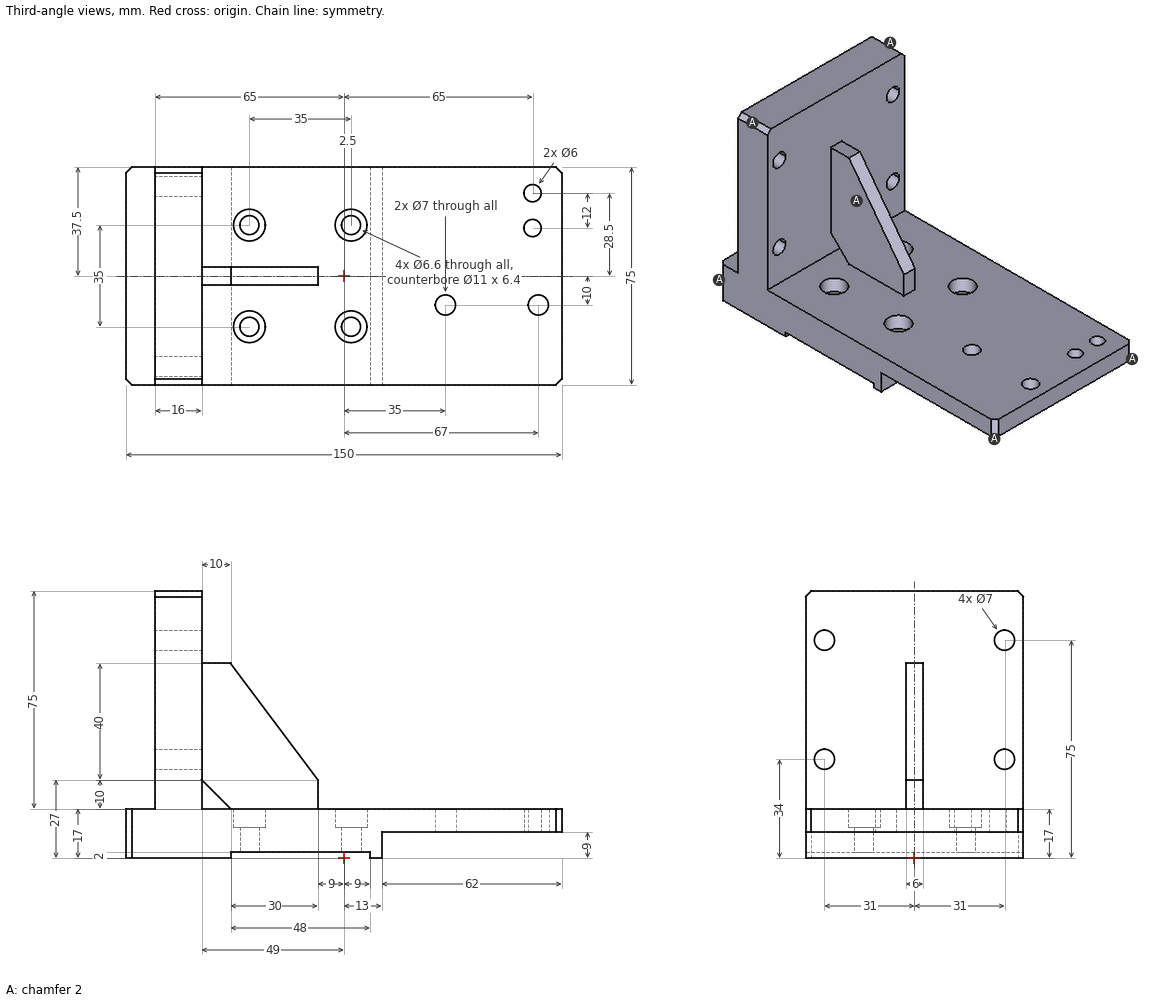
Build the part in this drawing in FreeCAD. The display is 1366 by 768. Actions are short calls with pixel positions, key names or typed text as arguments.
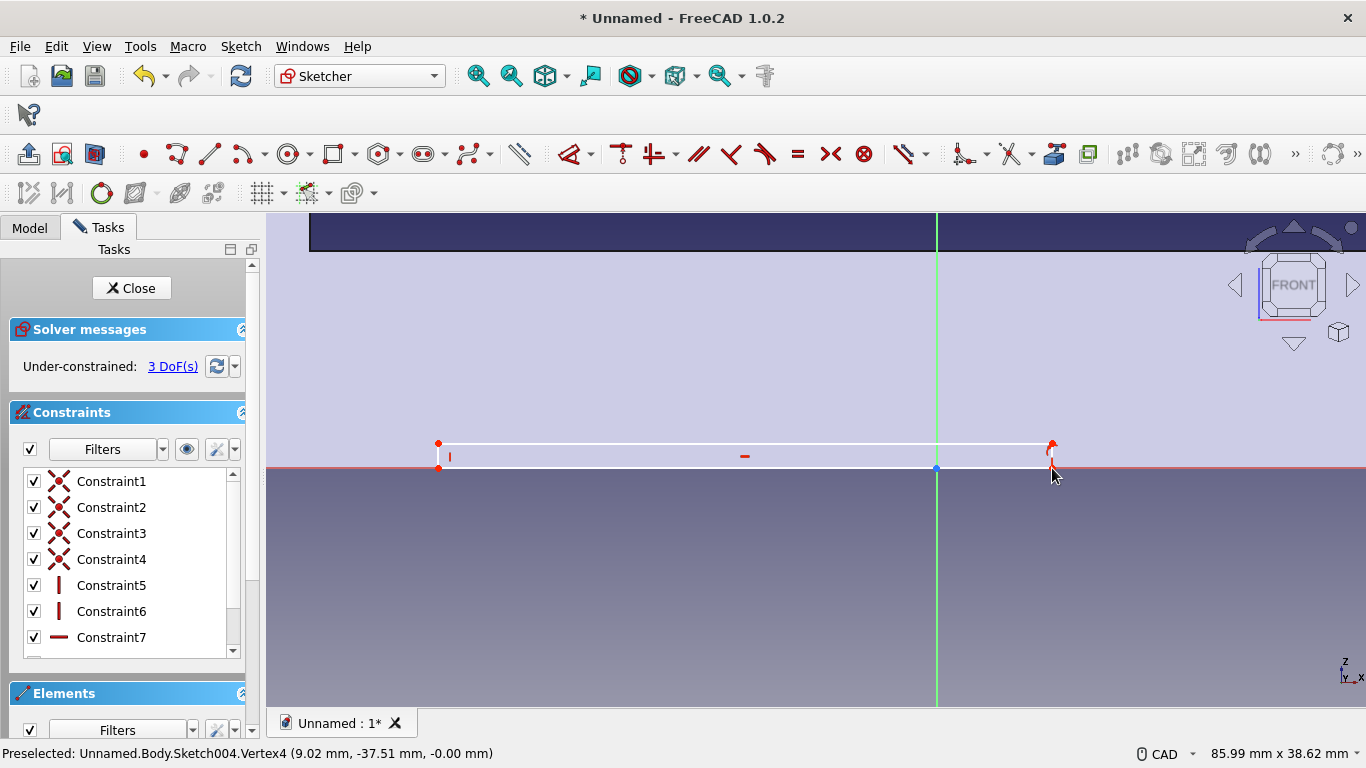
click(568, 154)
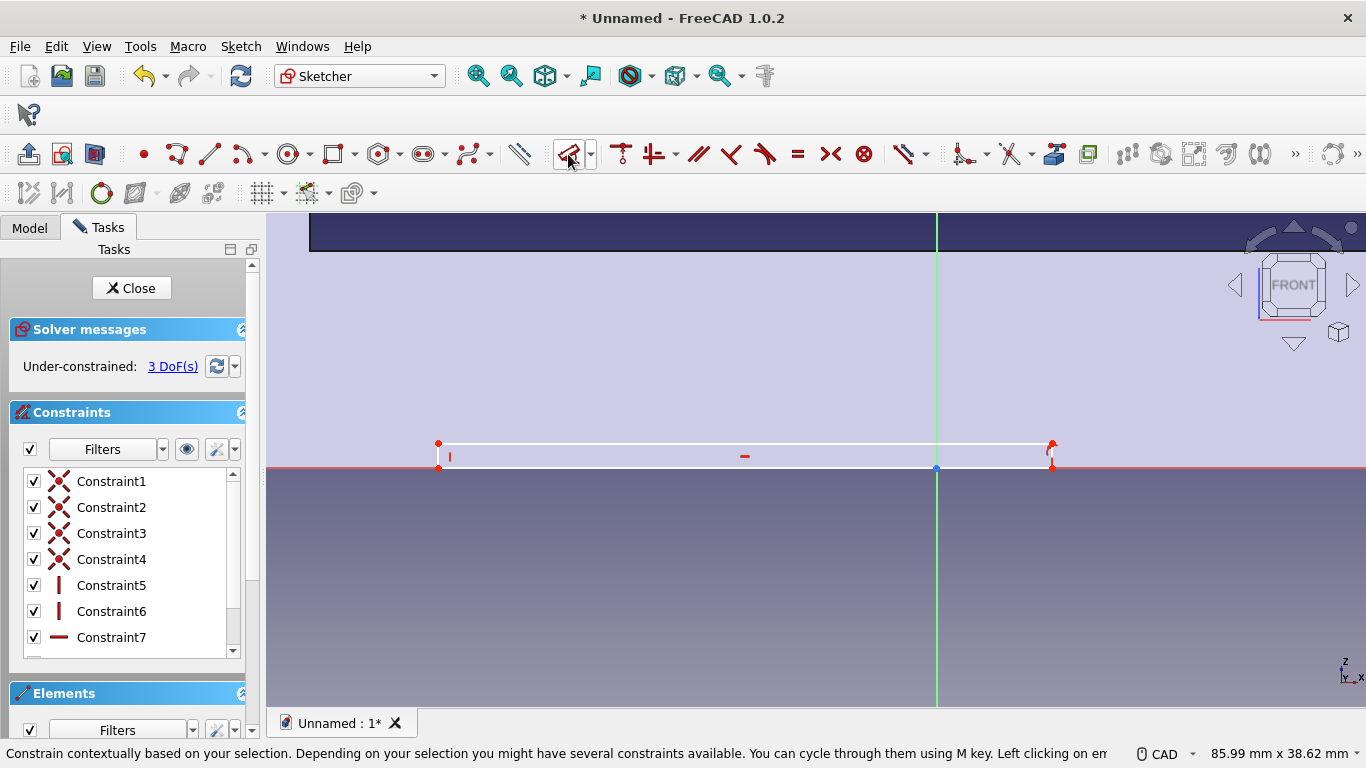
scroll(438, 454, up, 3)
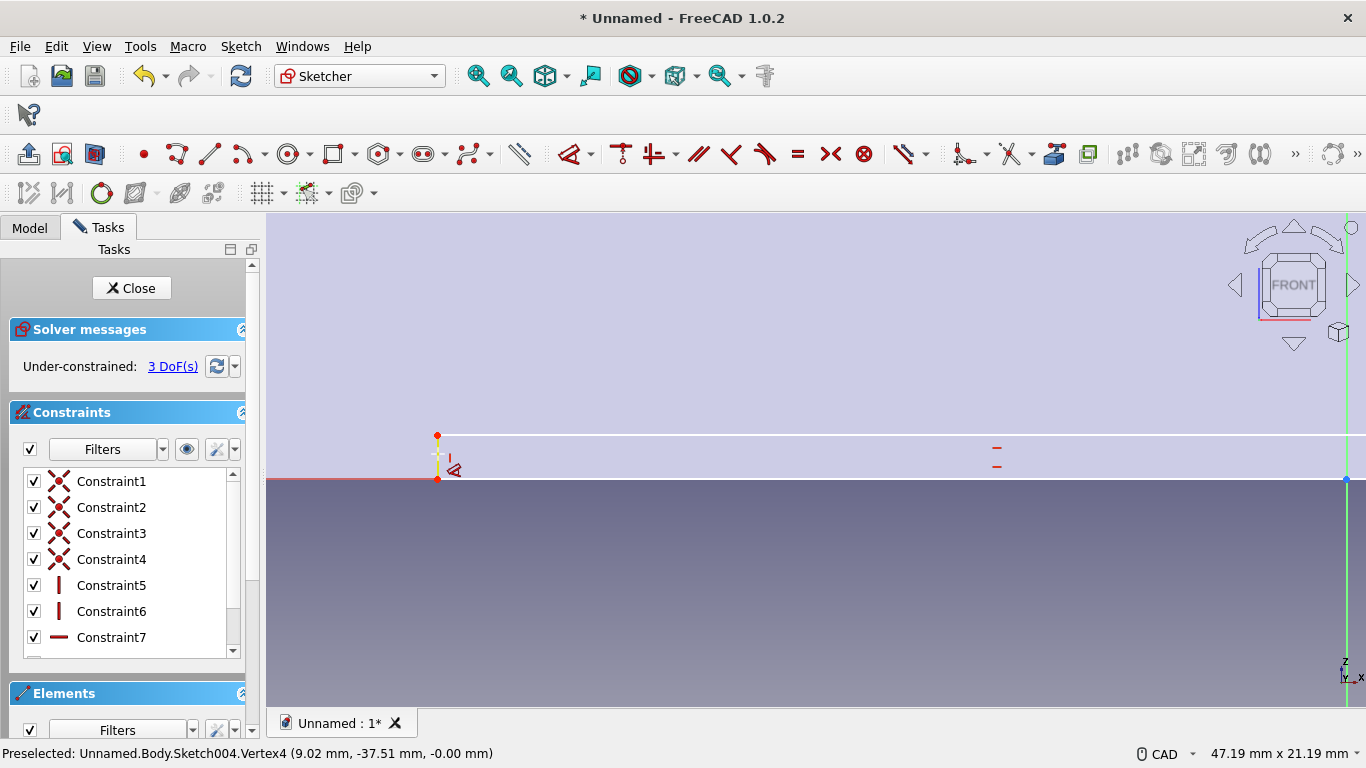
click(438, 453)
click(404, 457)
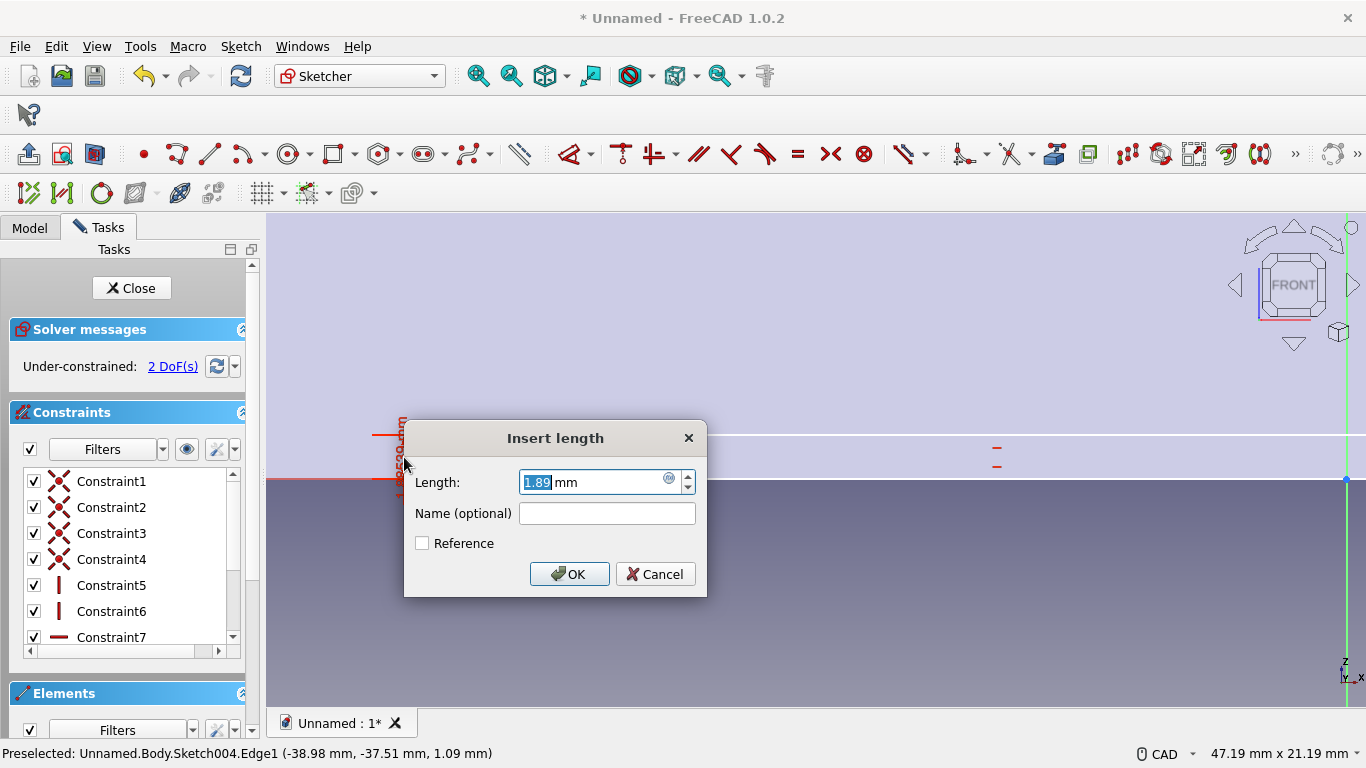
text(2)
key(Return)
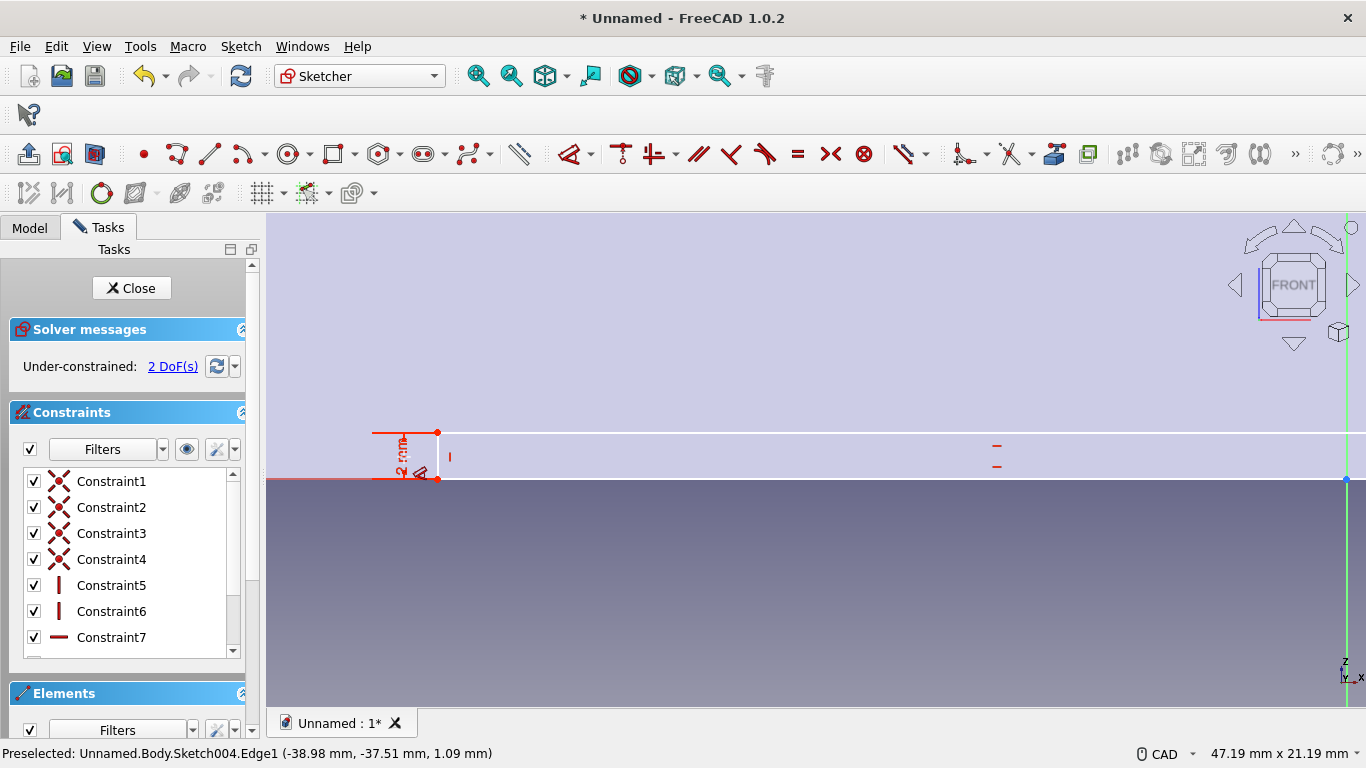
click(774, 479)
click(819, 513)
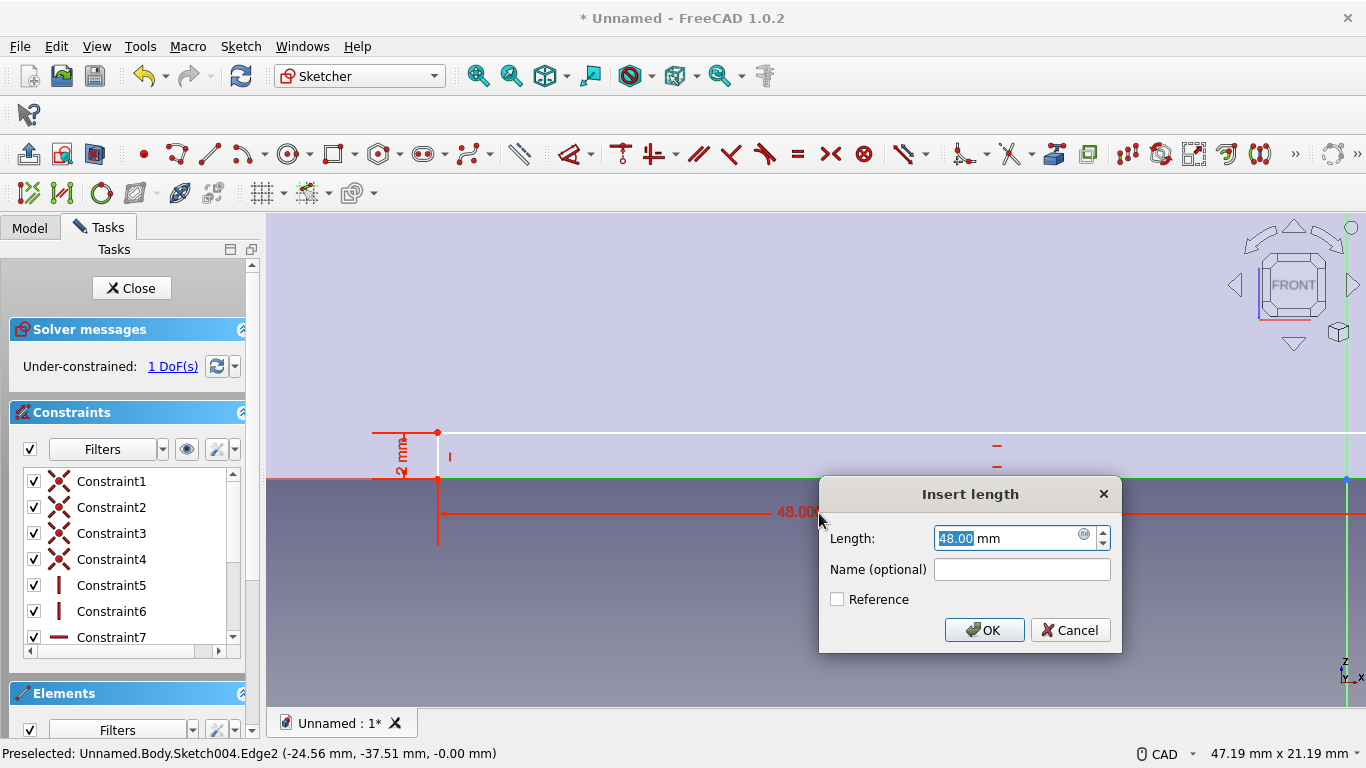
text(48)
key(Return)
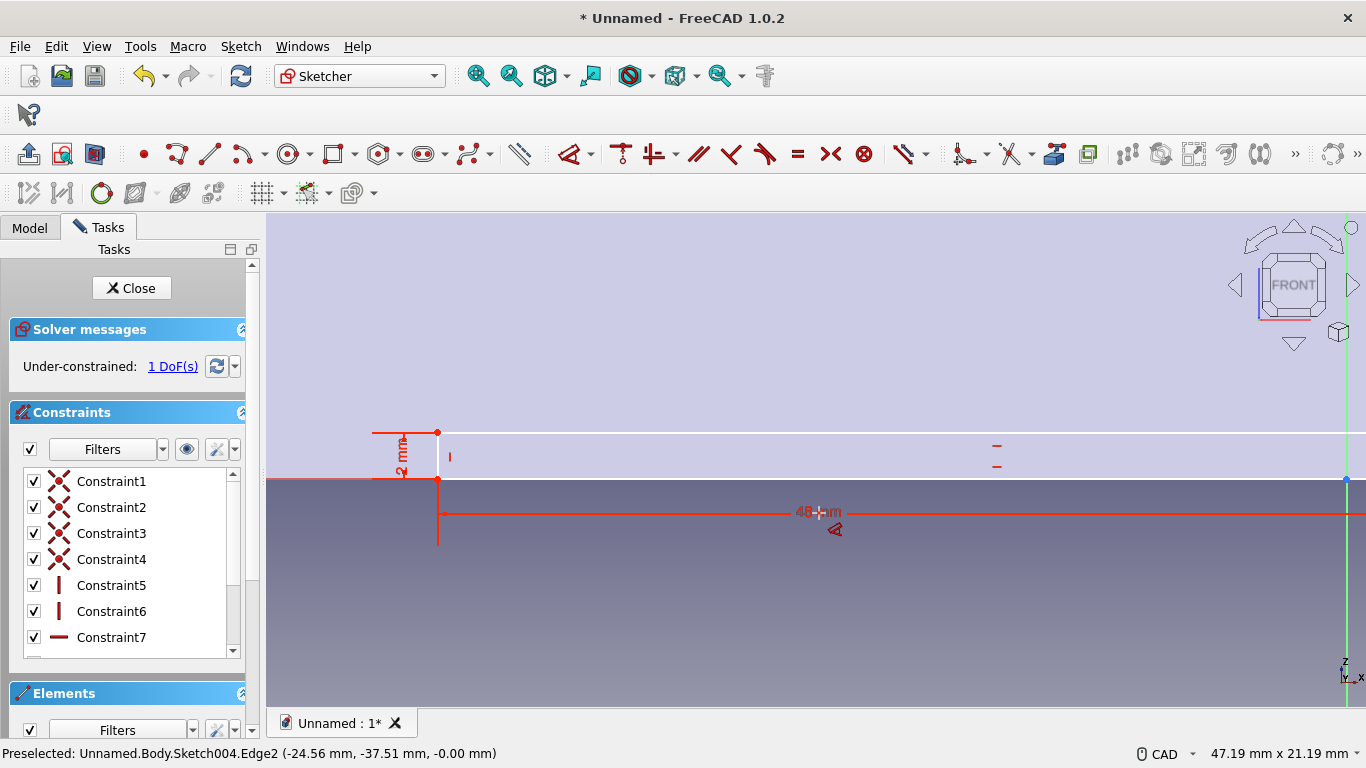
scroll(444, 465, down, 3)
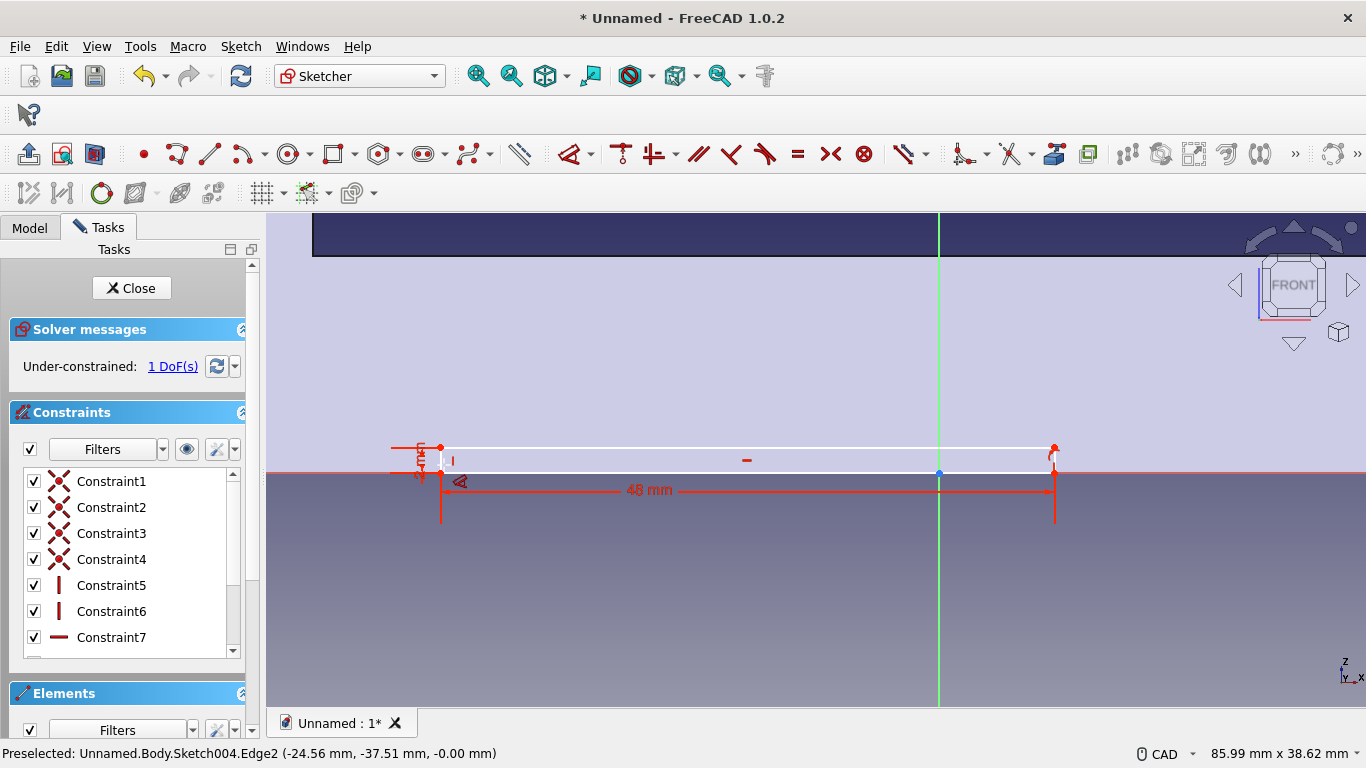
click(1055, 473)
click(997, 507)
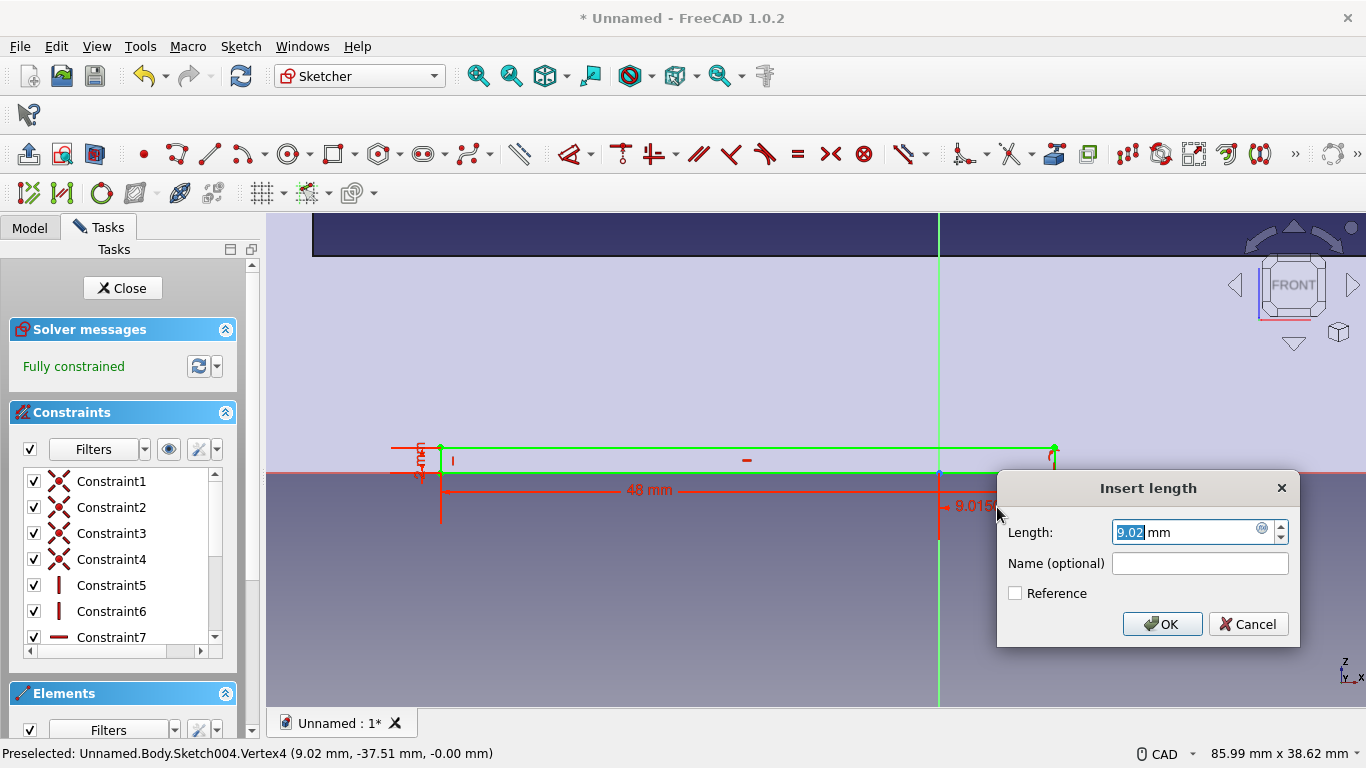
text(9)
key(Return)
key(Escape)